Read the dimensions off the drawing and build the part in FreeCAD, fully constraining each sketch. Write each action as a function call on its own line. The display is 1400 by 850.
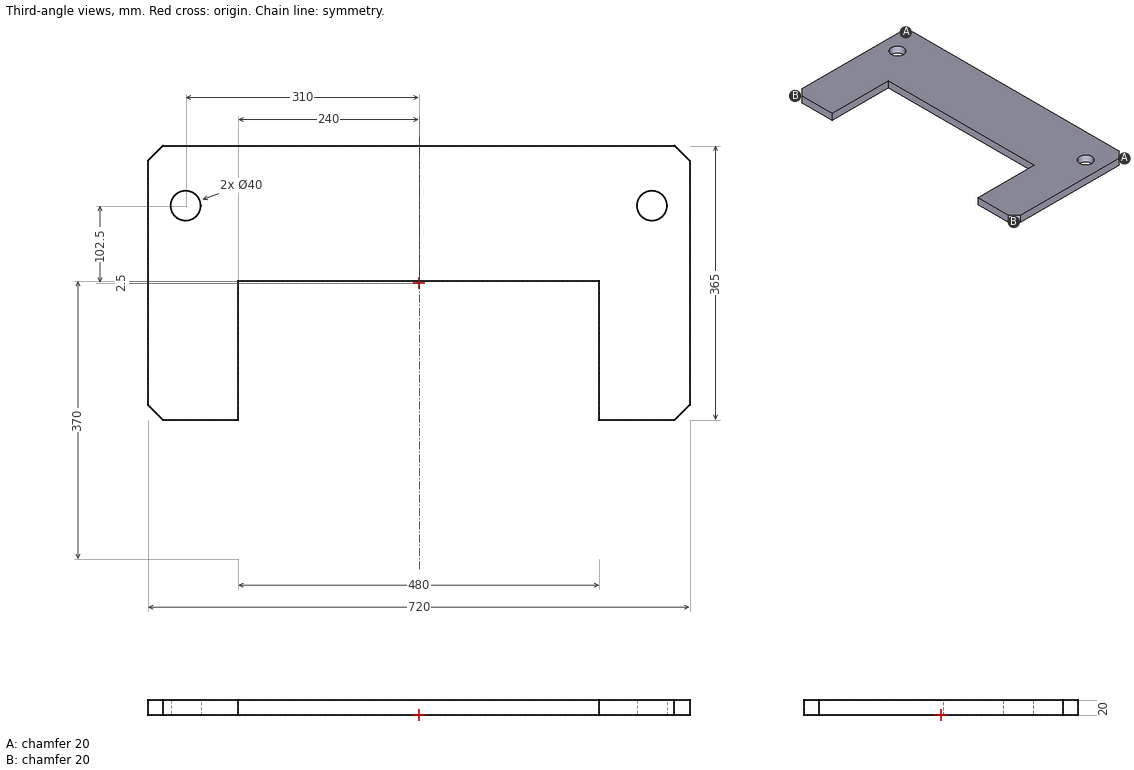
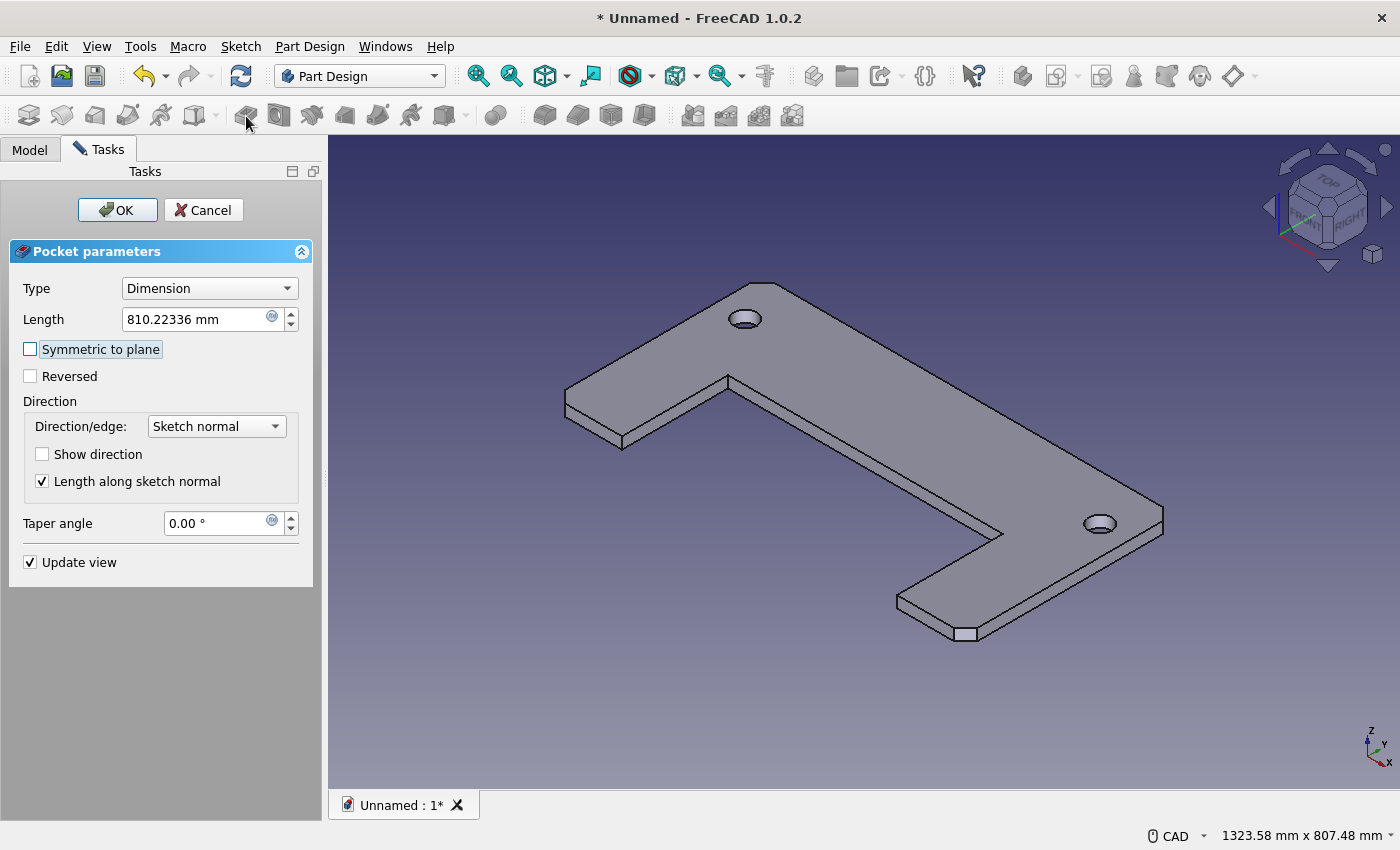
click(31, 349)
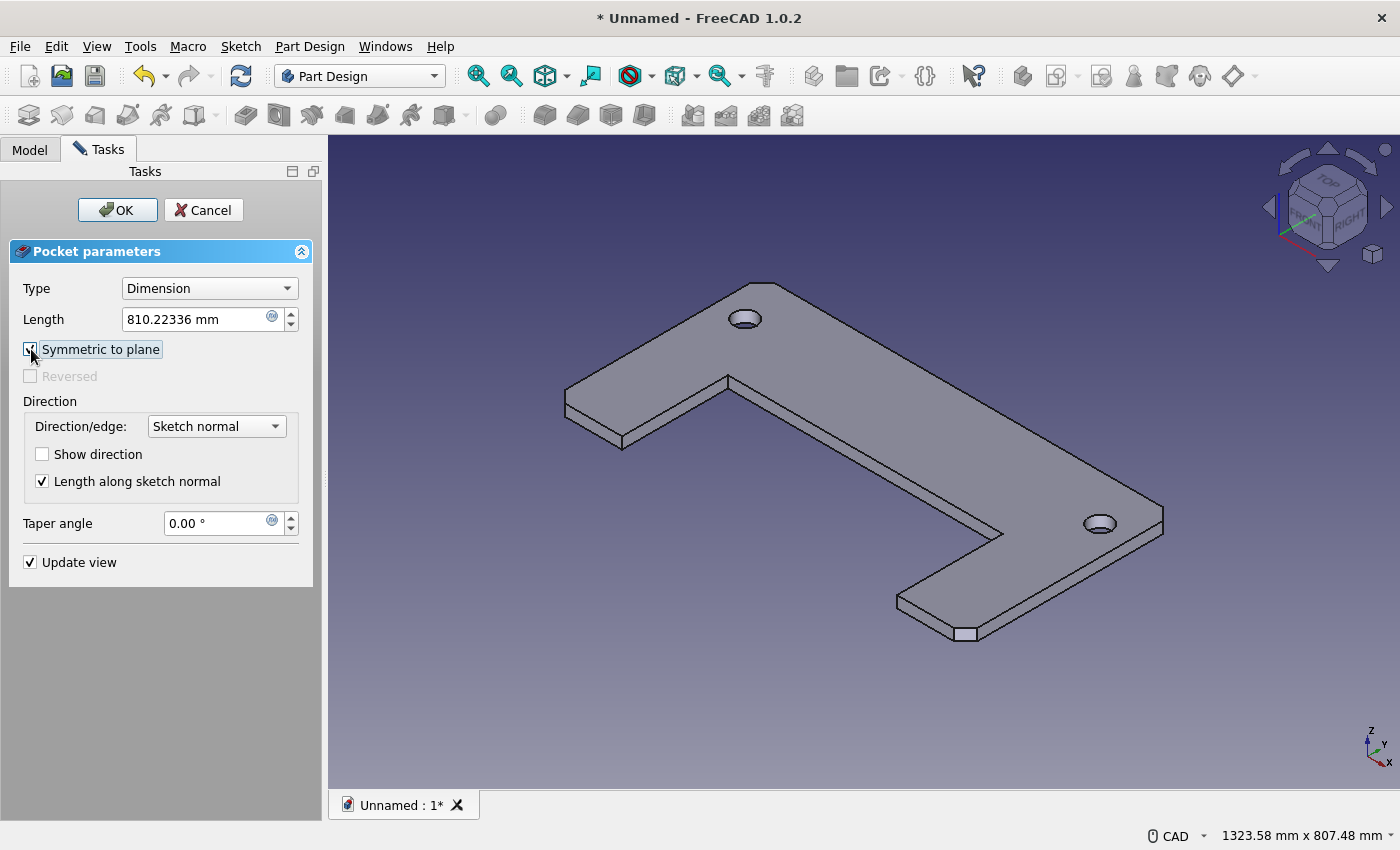
click(118, 210)